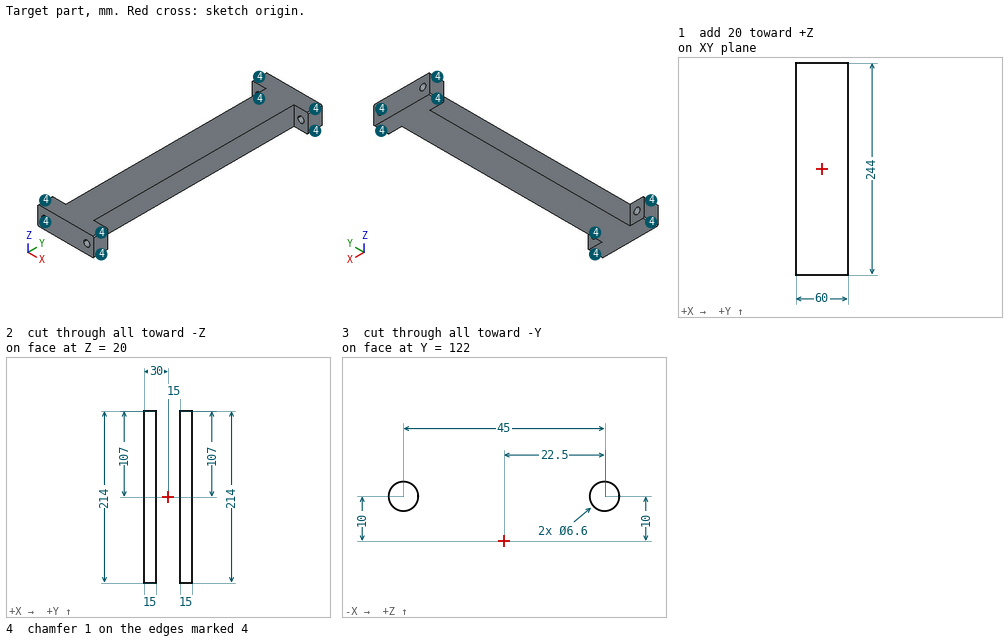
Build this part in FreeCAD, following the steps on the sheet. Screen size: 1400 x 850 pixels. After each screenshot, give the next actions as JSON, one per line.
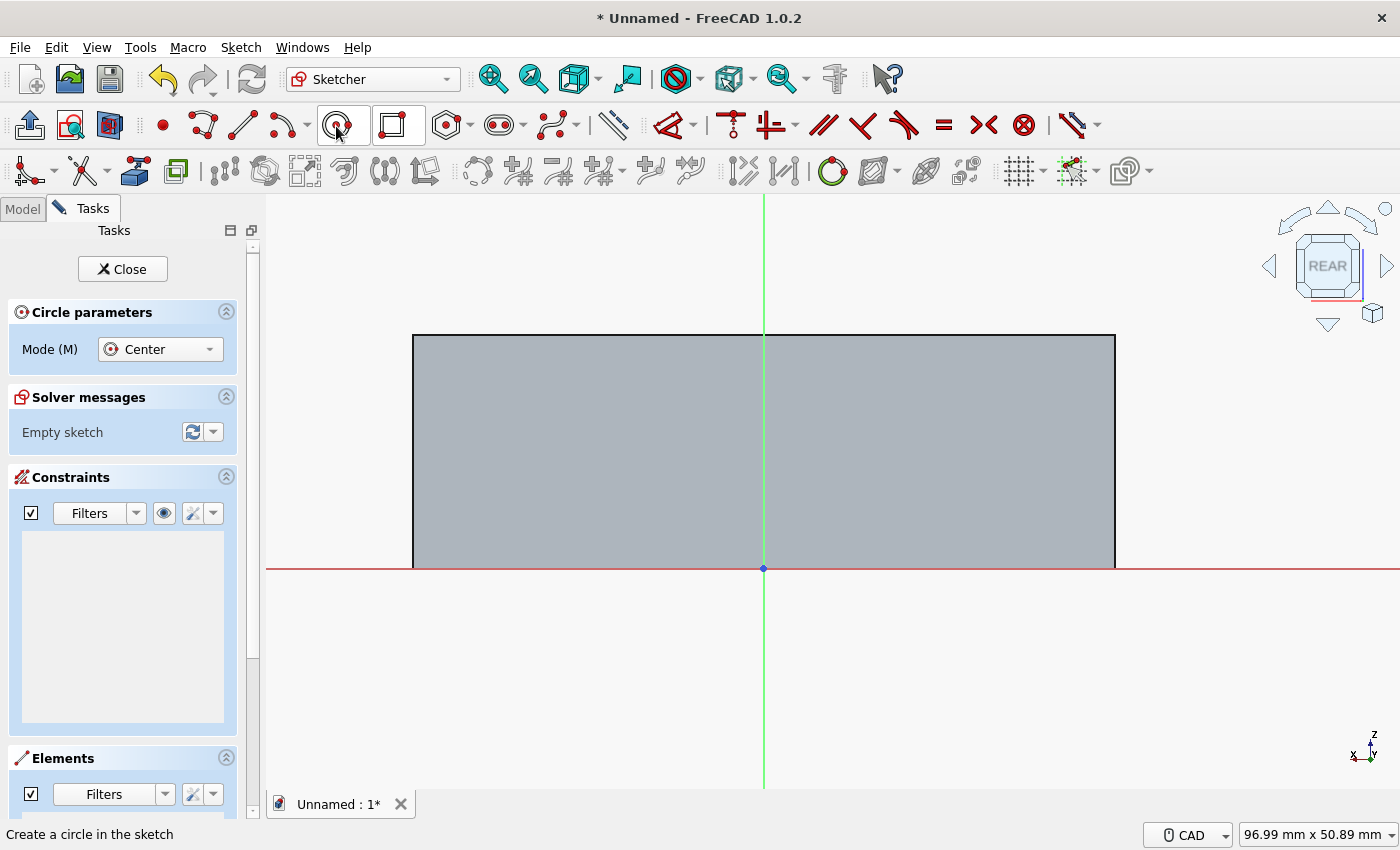
{"action": "left_click", "coordinate": [1027, 452]}
{"action": "mouse_move", "coordinate": [1054, 425]}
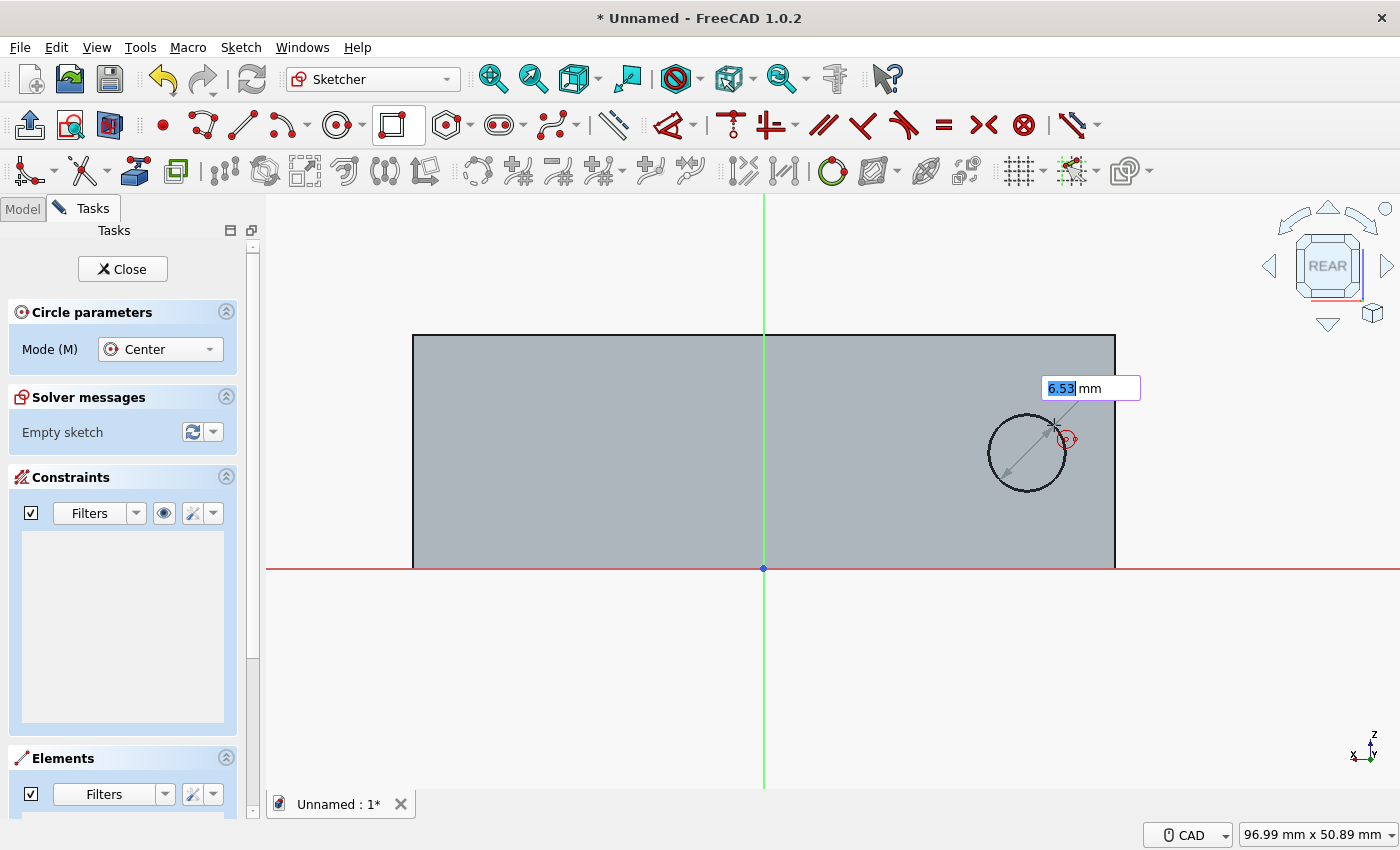
{"action": "type", "text": "6.6"}
{"action": "key", "text": "Return"}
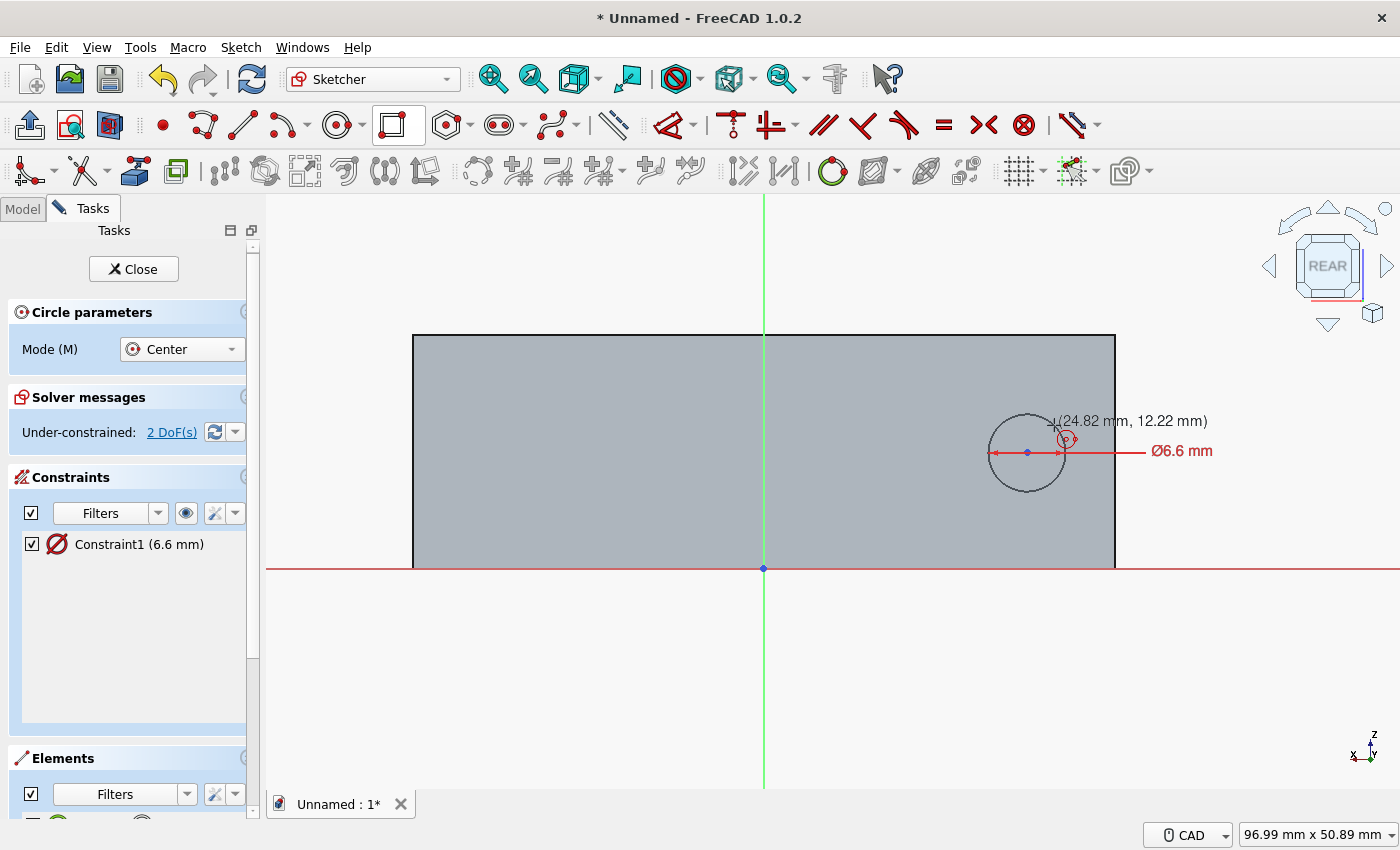
{"action": "left_click", "coordinate": [501, 452]}
{"action": "mouse_move", "coordinate": [528, 425]}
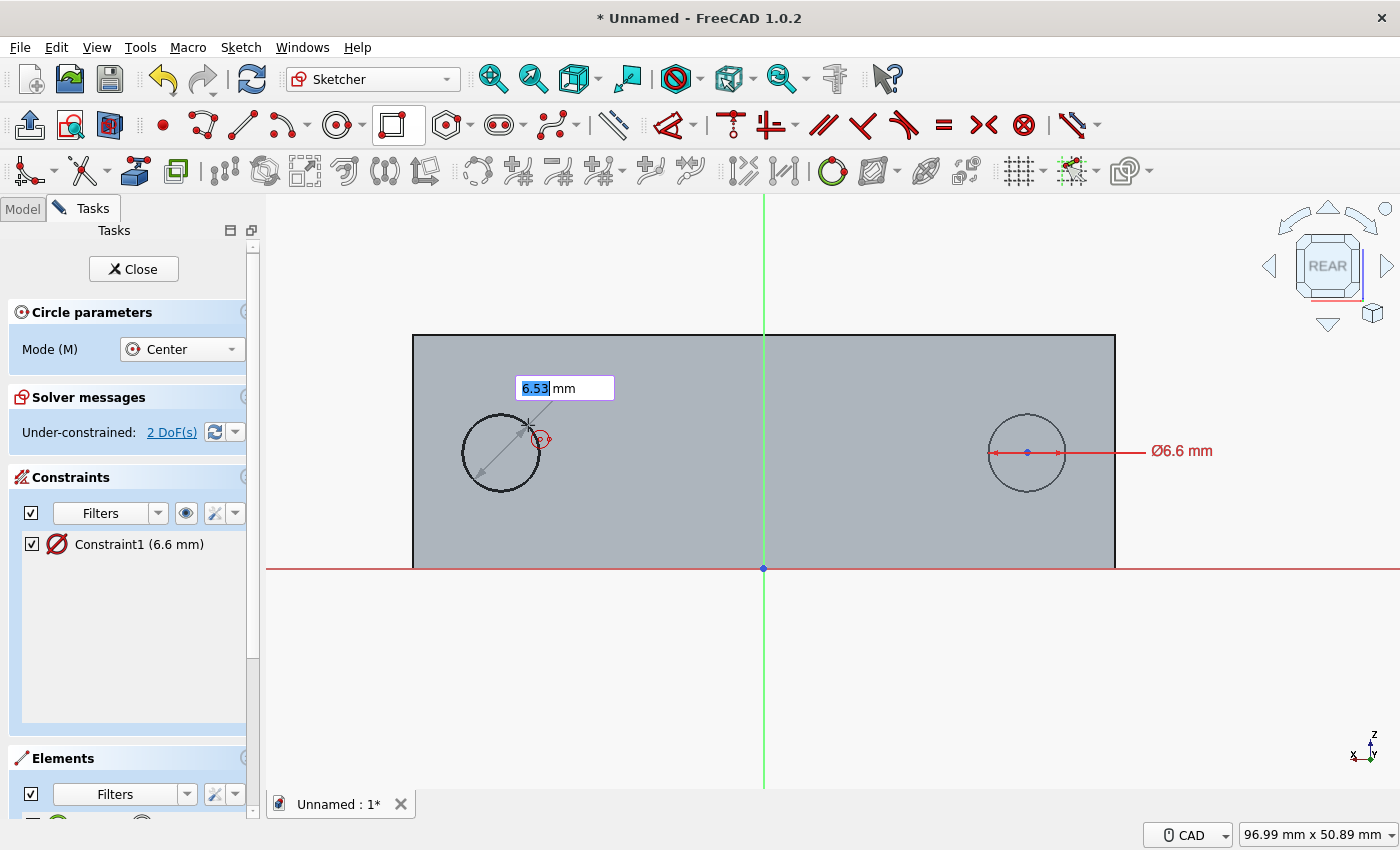
{"action": "type", "text": "6.6"}
{"action": "key", "text": "Return"}
{"action": "key", "text": "Escape"}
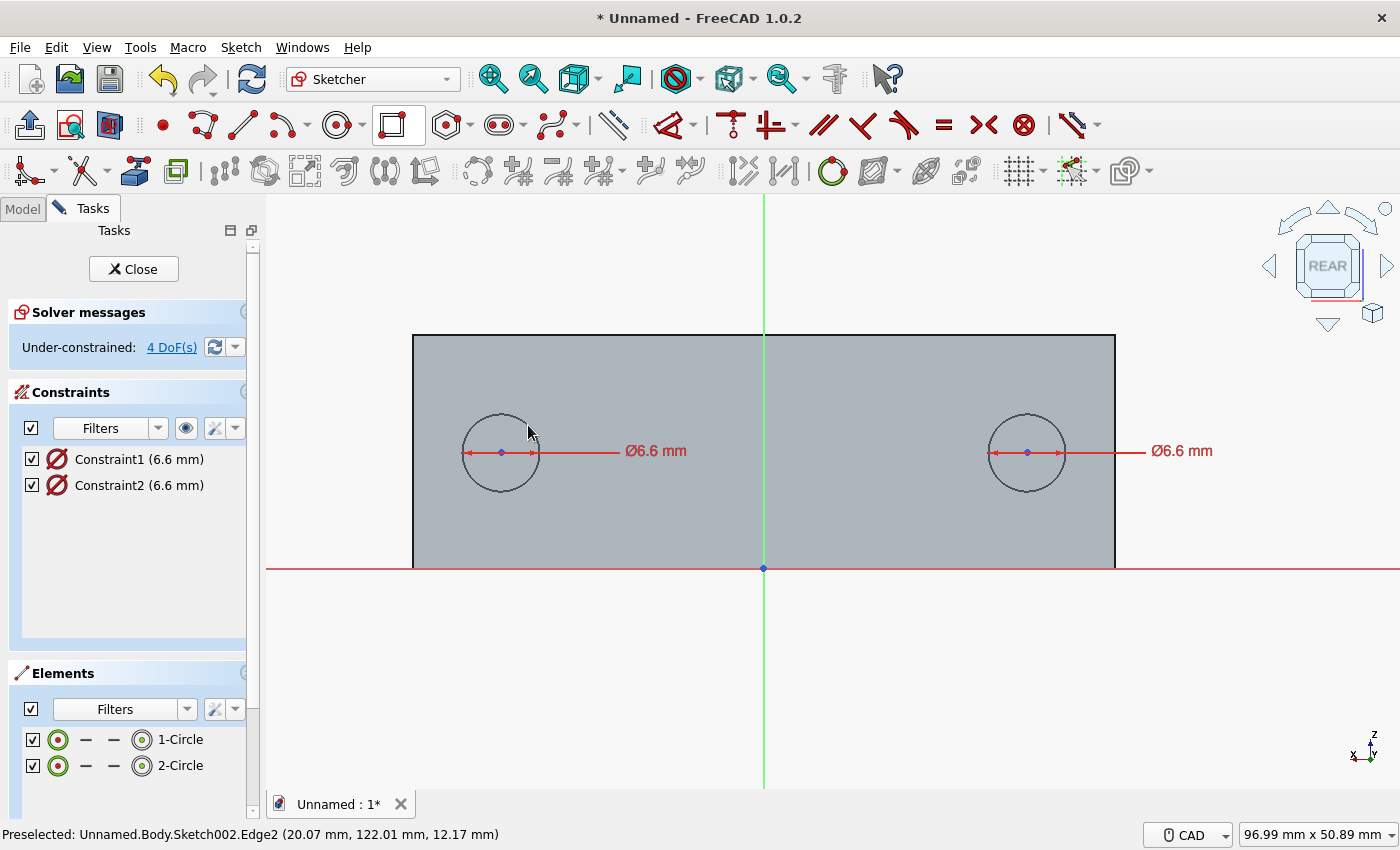
{"action": "left_click", "coordinate": [668, 126]}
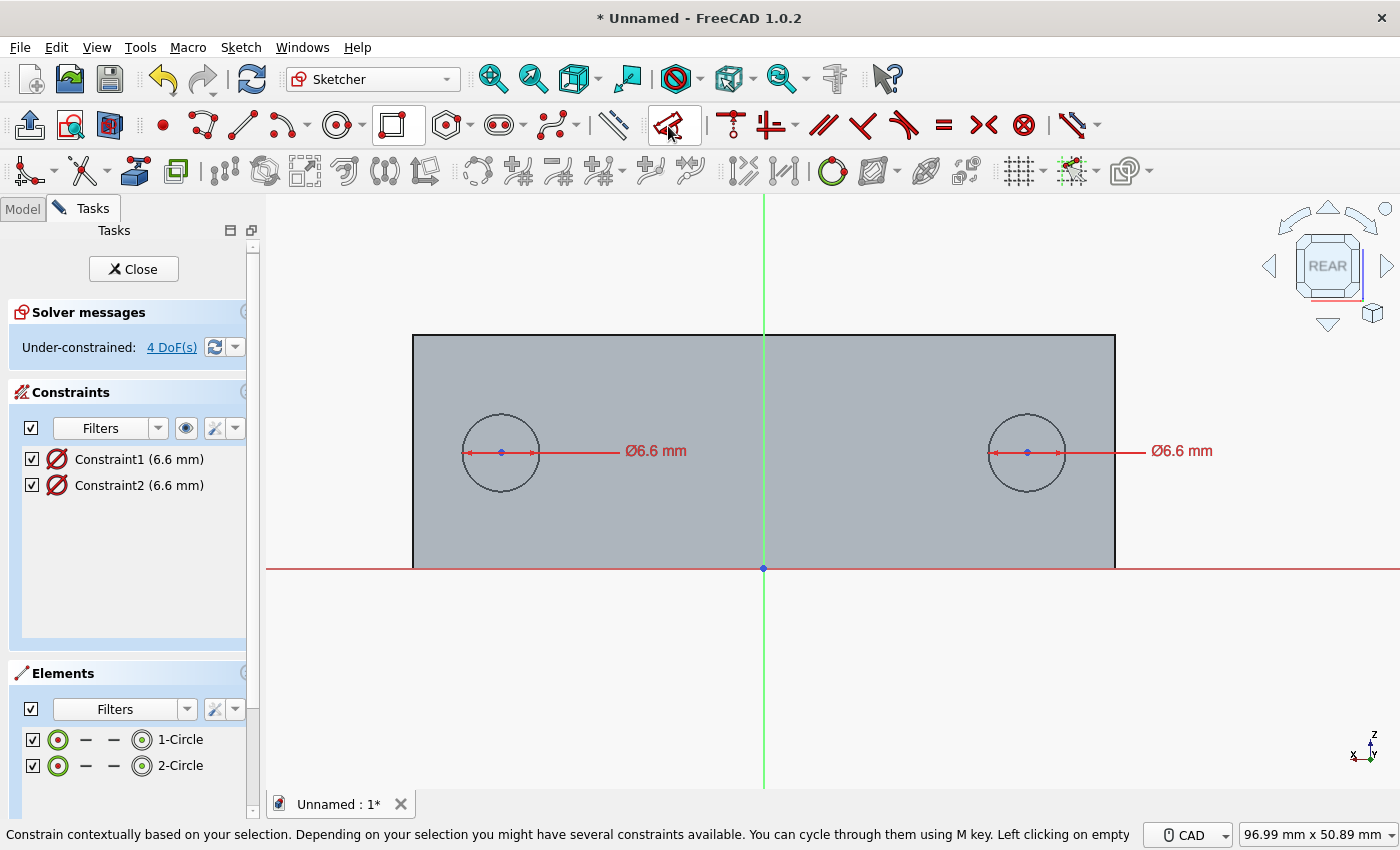
{"action": "left_click", "coordinate": [1027, 453]}
{"action": "left_click", "coordinate": [1061, 511]}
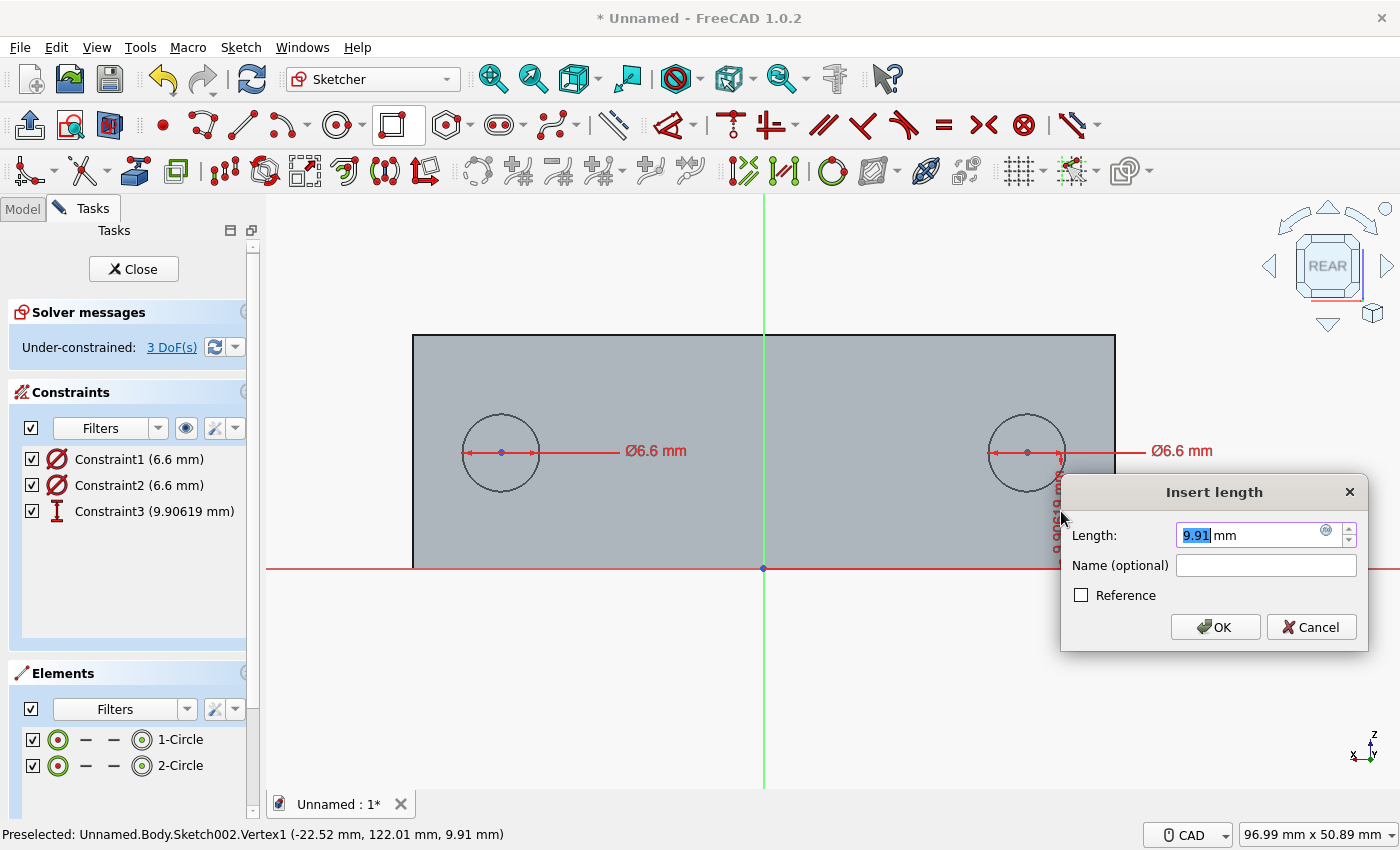
{"action": "type", "text": "10"}
{"action": "key", "text": "Return"}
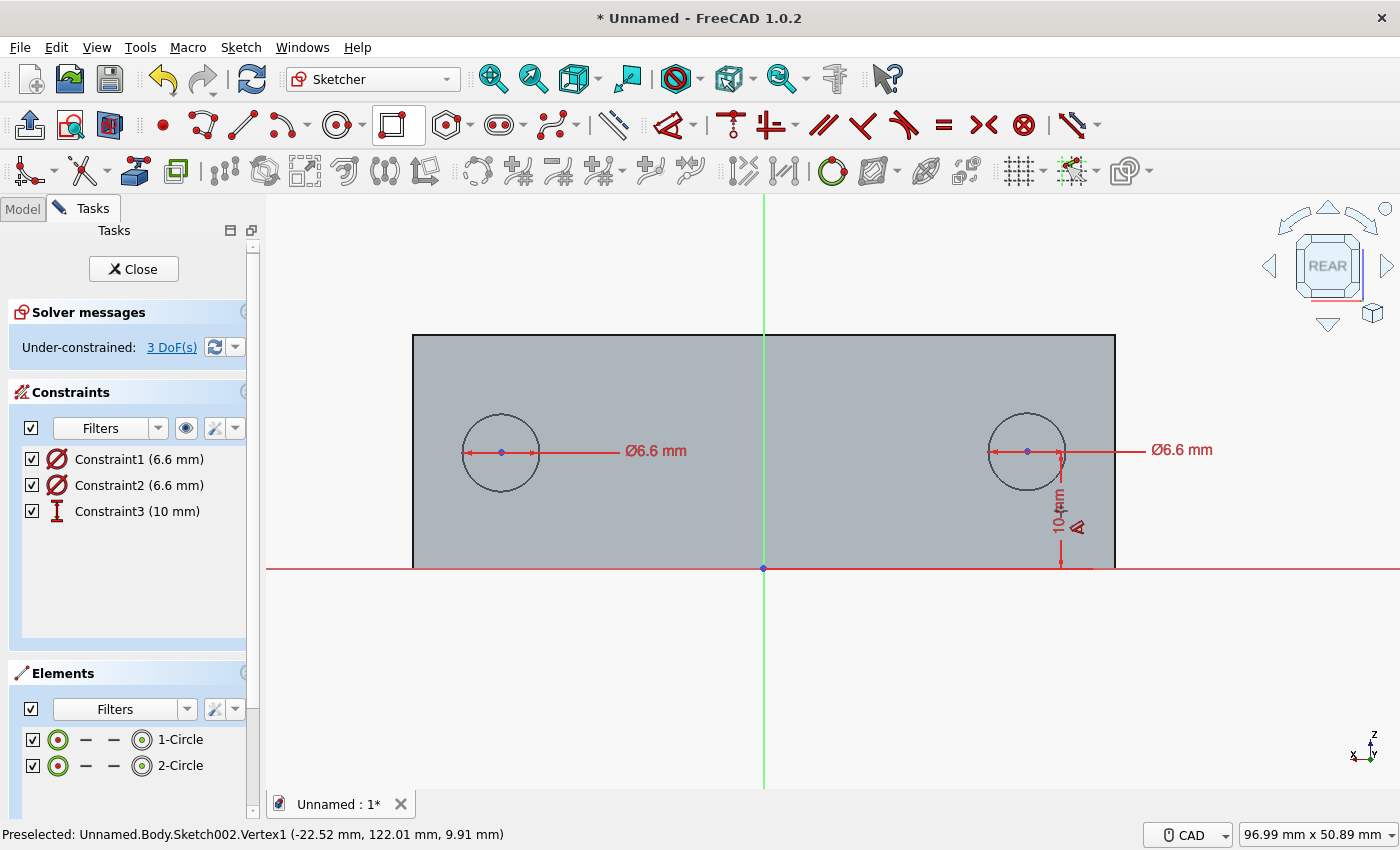
{"action": "left_click", "coordinate": [501, 453]}
{"action": "left_click", "coordinate": [467, 511]}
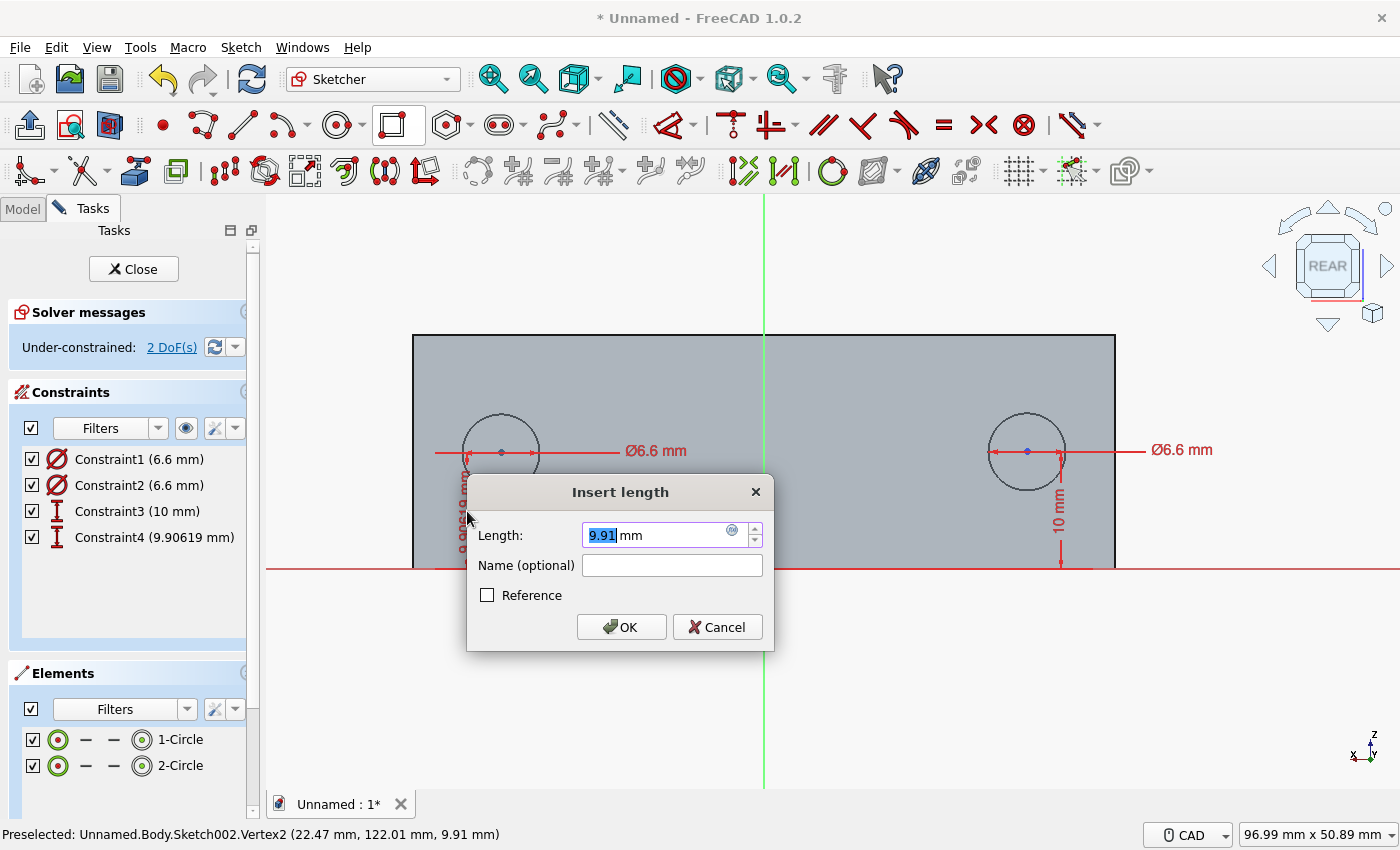
{"action": "type", "text": "10"}
{"action": "key", "text": "Return"}